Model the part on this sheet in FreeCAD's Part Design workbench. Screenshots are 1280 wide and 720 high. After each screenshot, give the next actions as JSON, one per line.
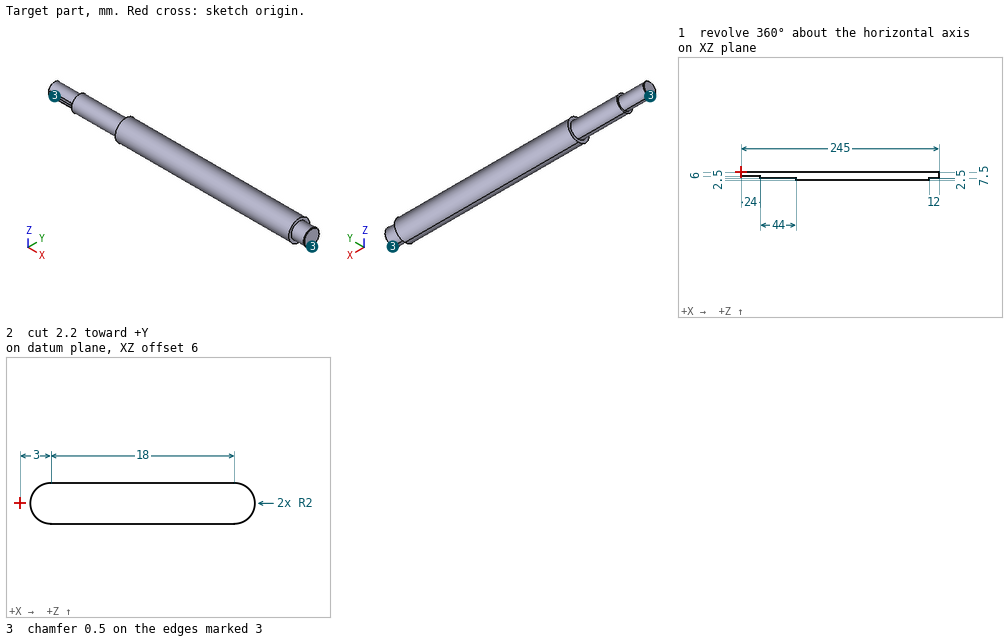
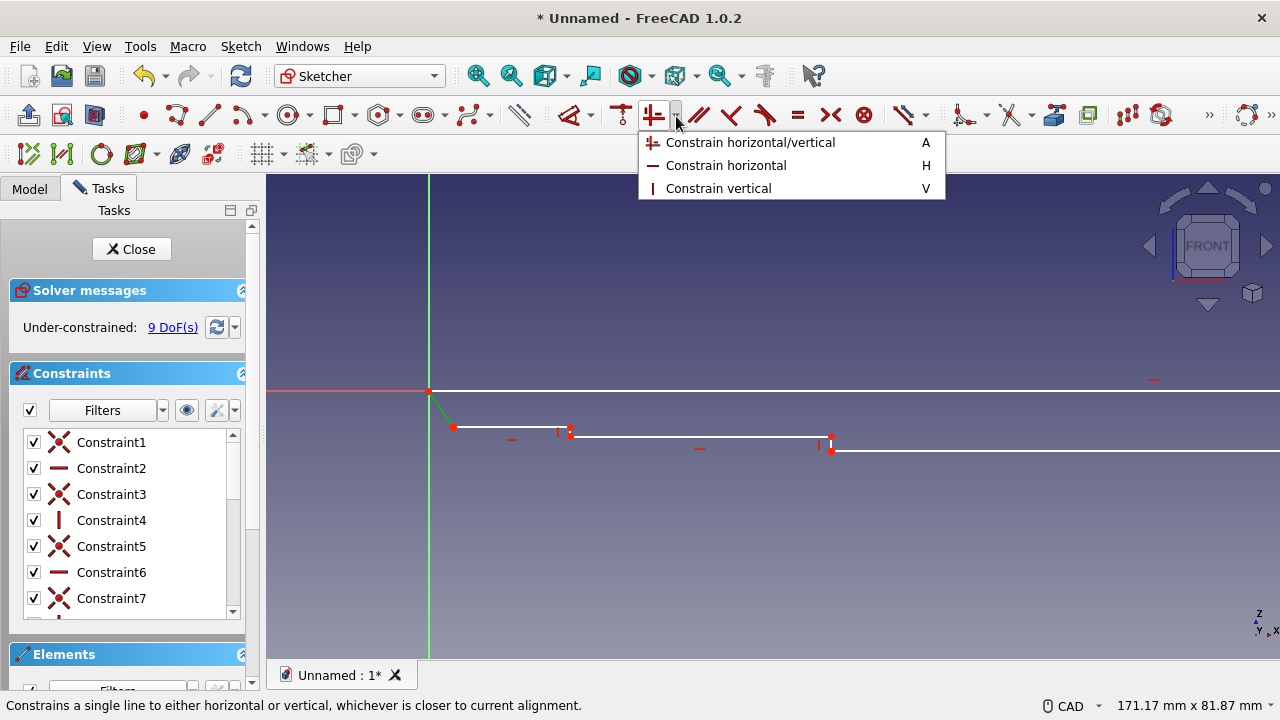
{"action": "left_click", "coordinate": [792, 188]}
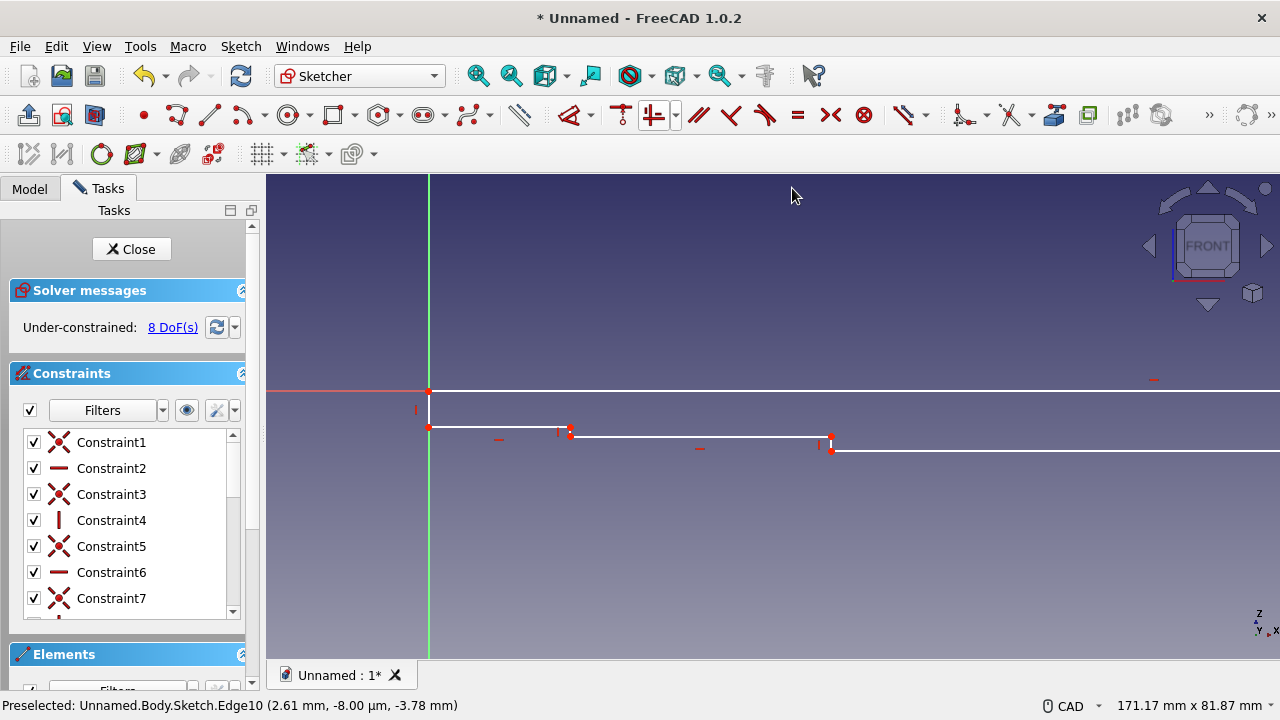
{"action": "scroll", "coordinate": [429, 417], "scroll_direction": "up", "scroll_amount": 2}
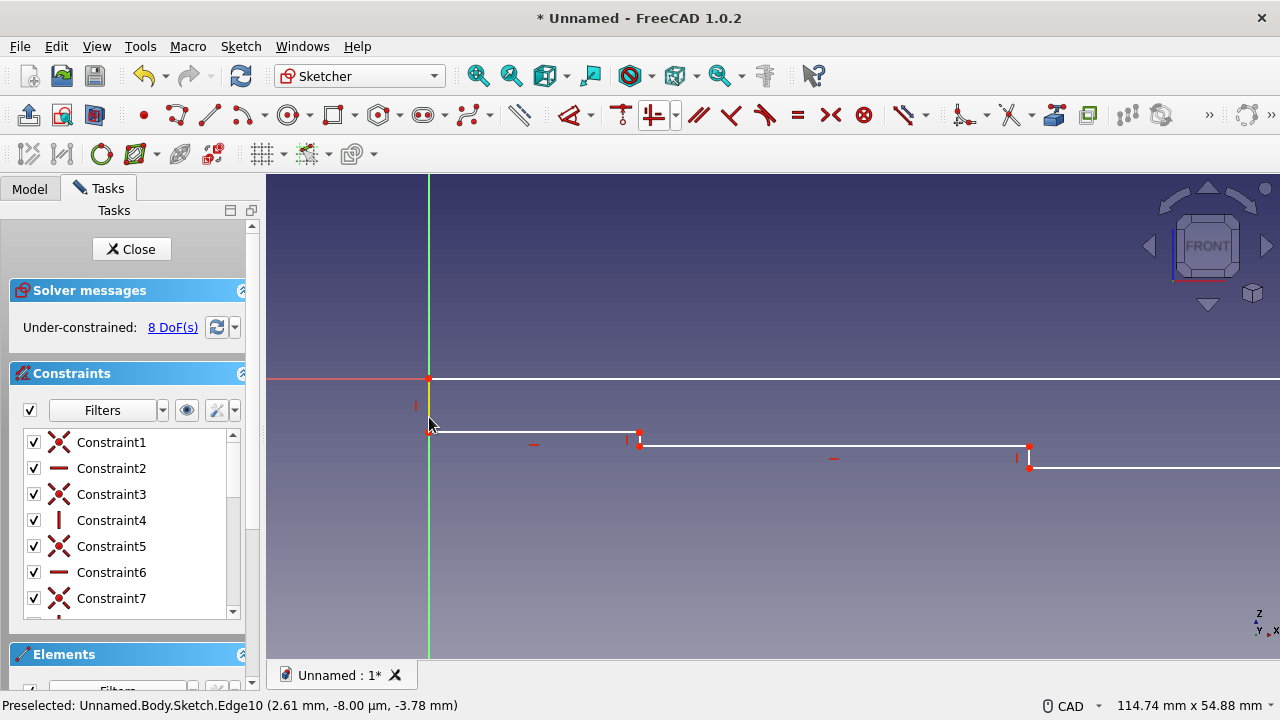
{"action": "left_click", "coordinate": [429, 416]}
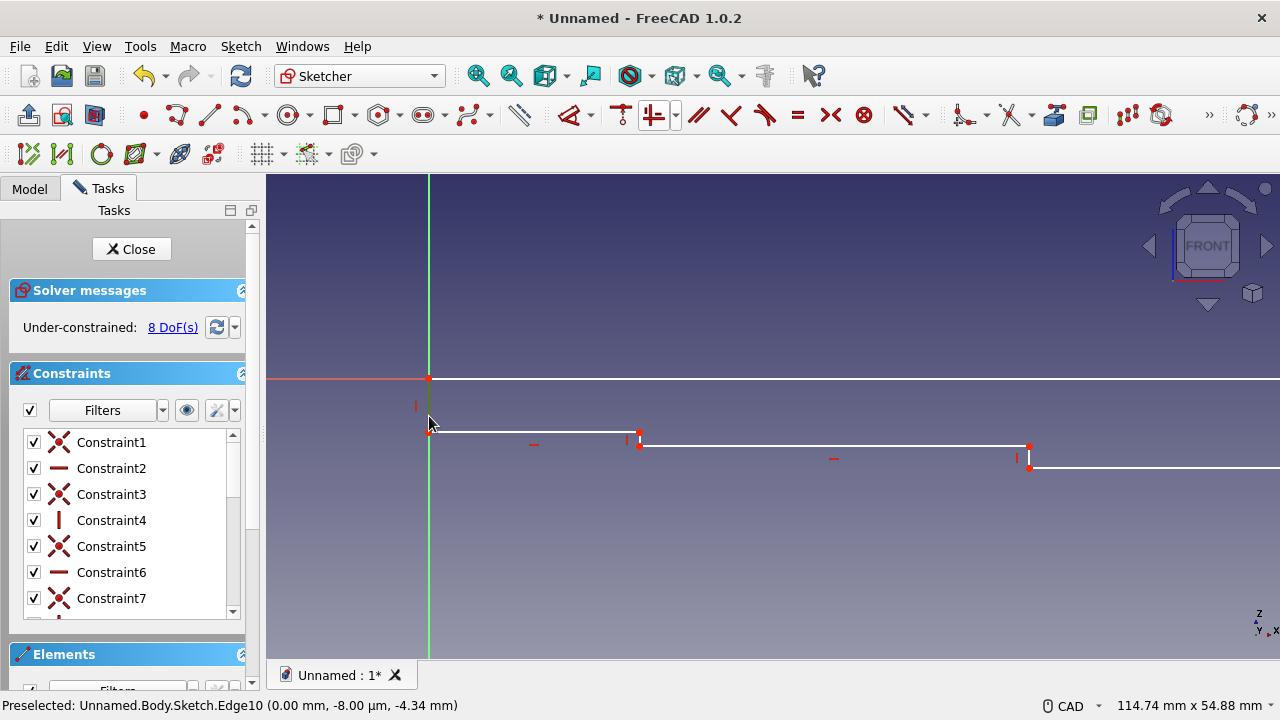
{"action": "key", "text": "i"}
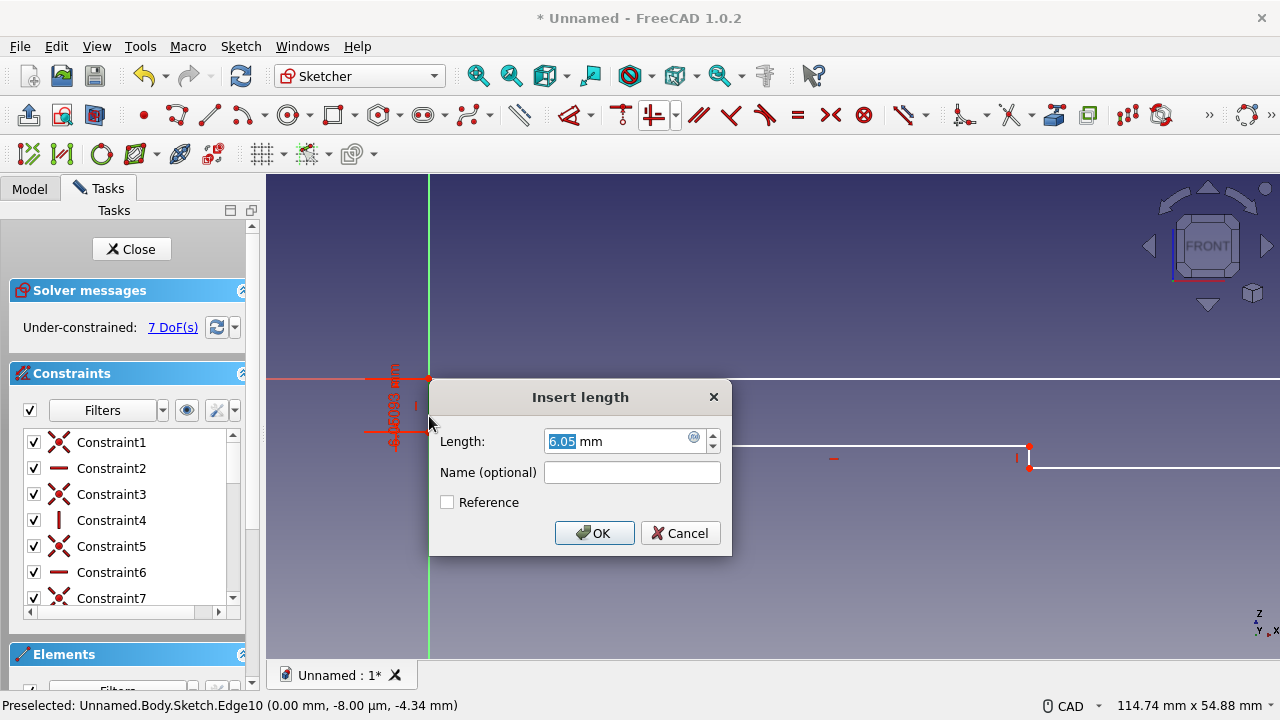
{"action": "type", "text": "6"}
{"action": "key", "text": "Return"}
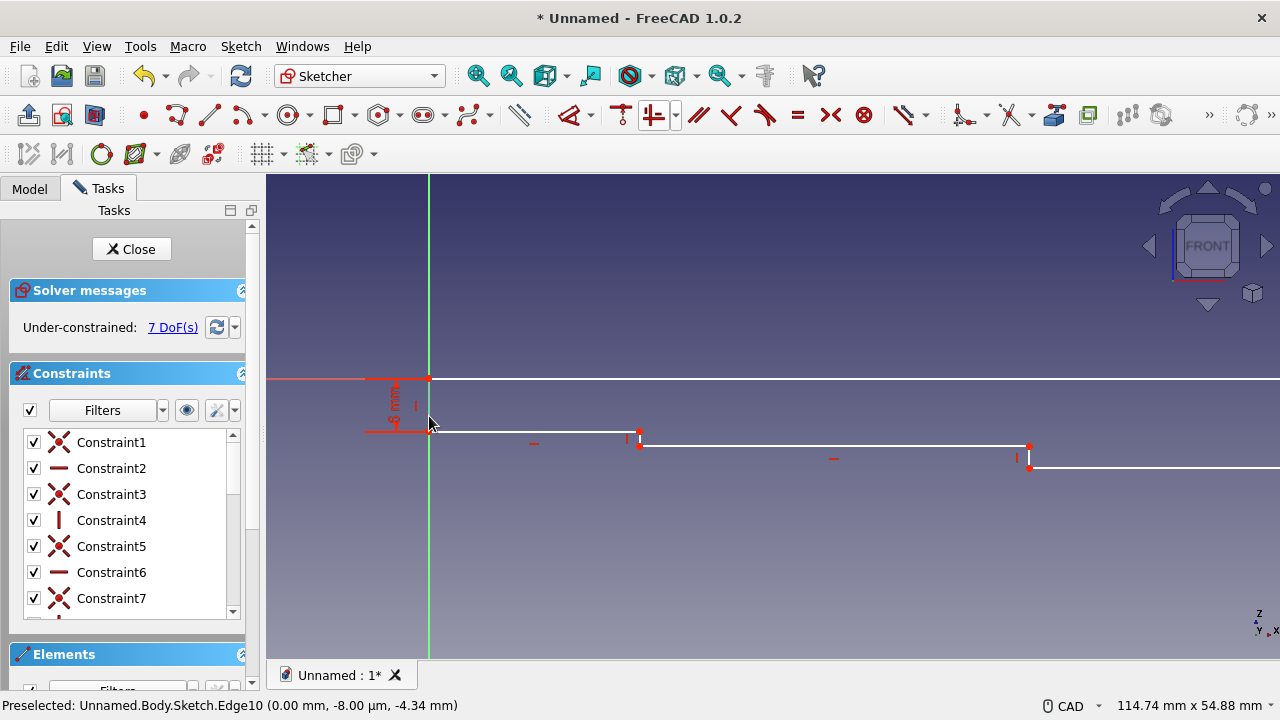
{"action": "scroll", "coordinate": [440, 414], "scroll_direction": "down", "scroll_amount": 7}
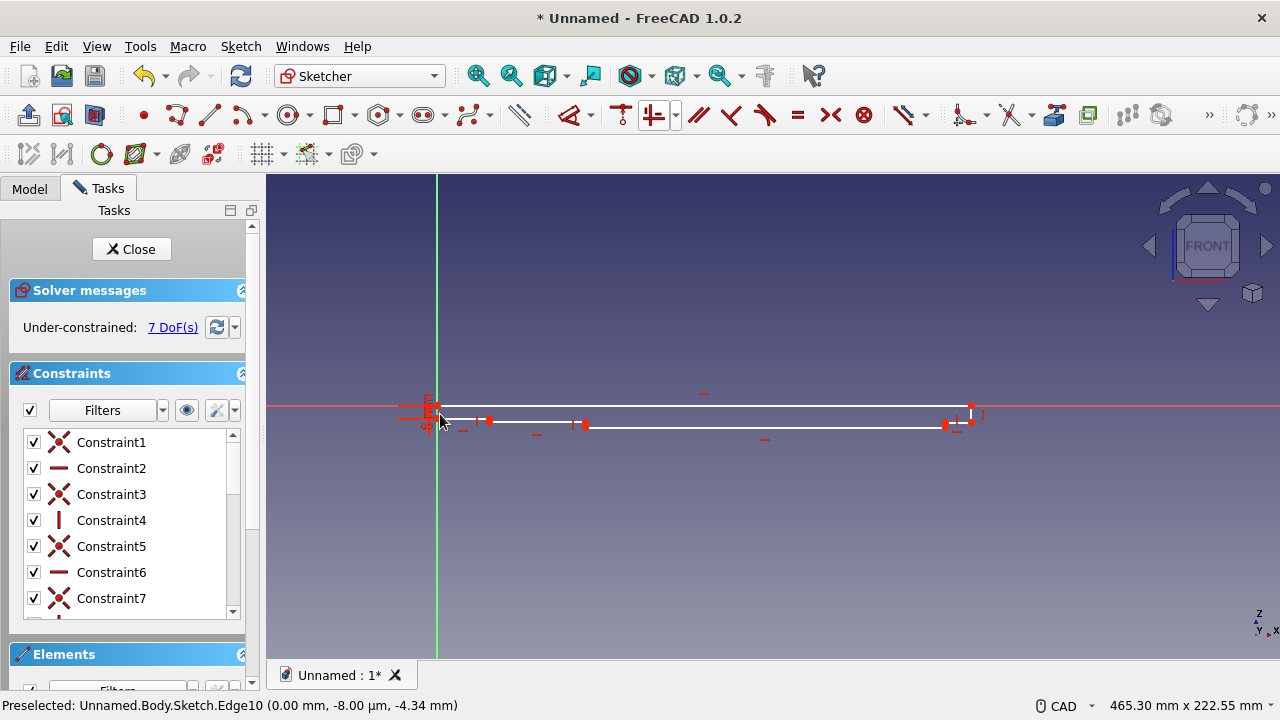
{"action": "scroll", "coordinate": [963, 423], "scroll_direction": "up", "scroll_amount": 3}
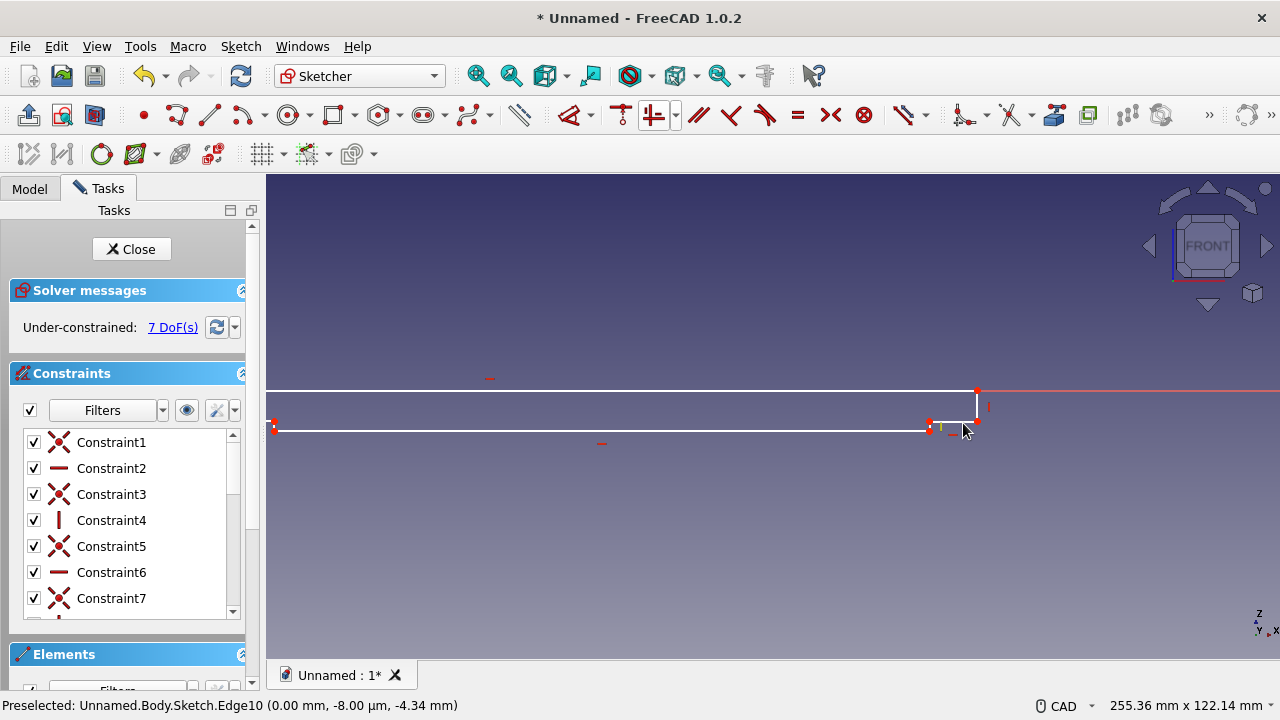
{"action": "left_click", "coordinate": [963, 422]}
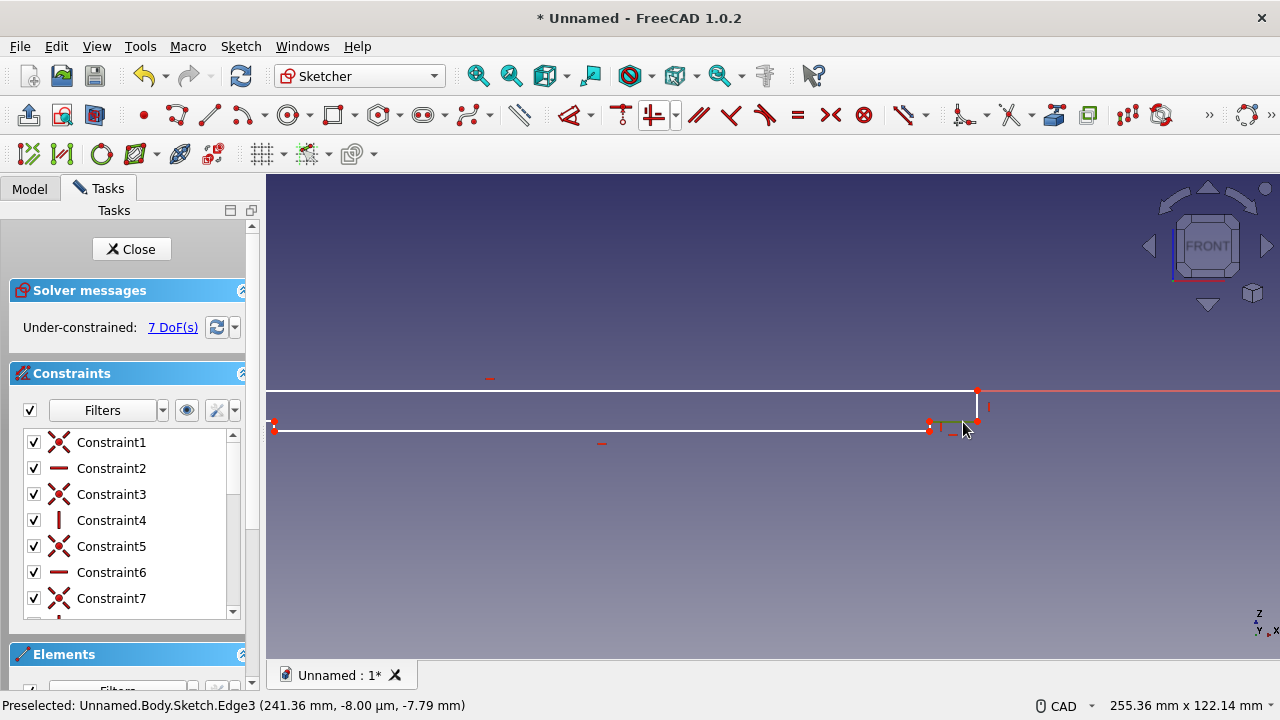
{"action": "key", "text": "l"}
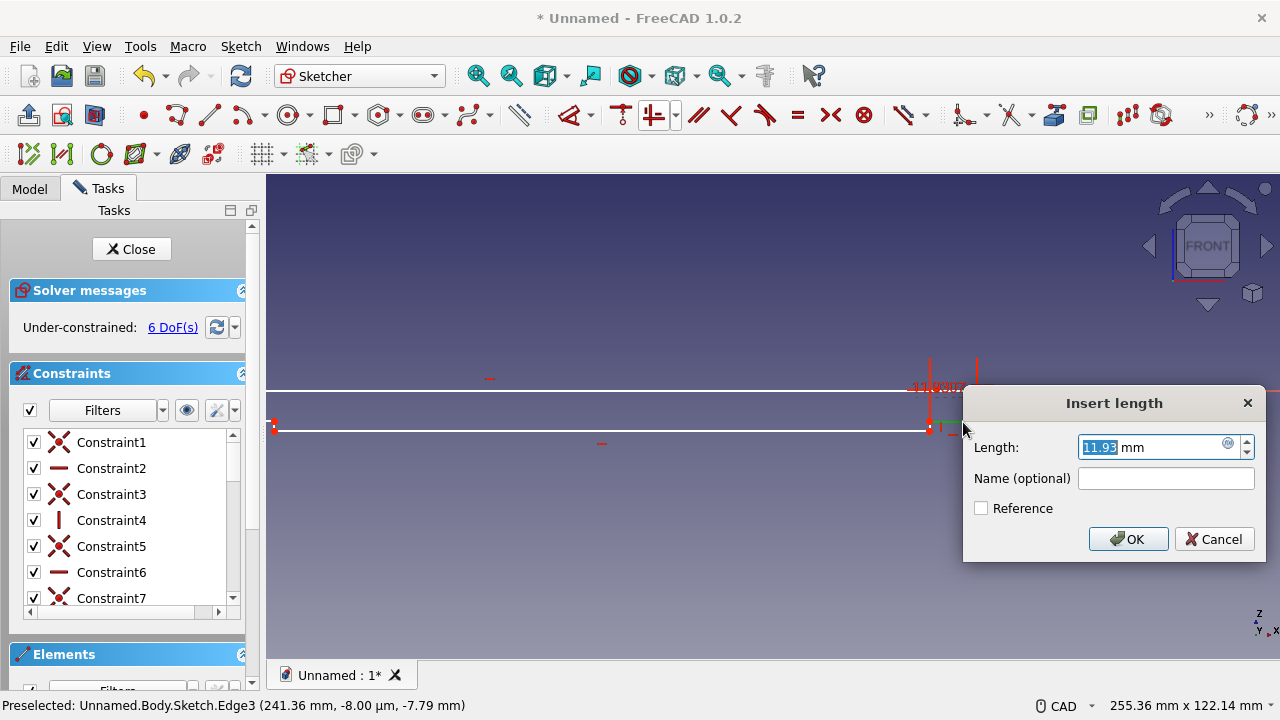
{"action": "type", "text": "12"}
{"action": "key", "text": "Return"}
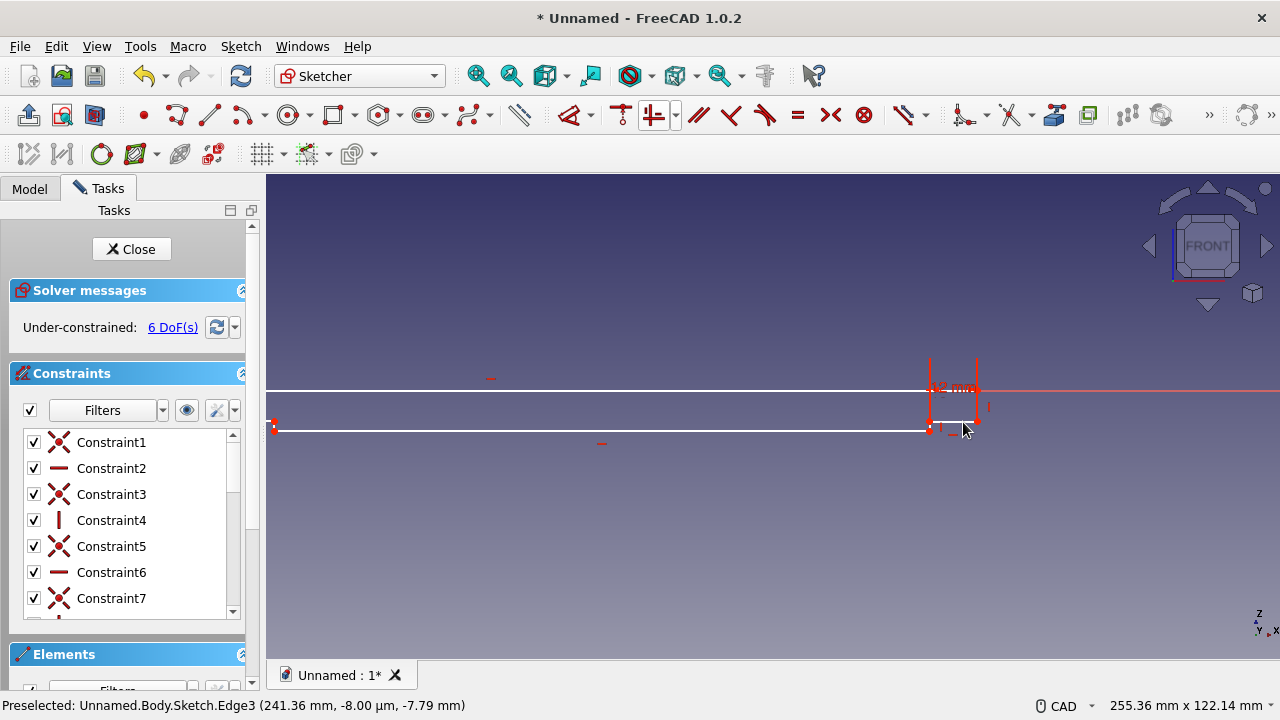
{"action": "scroll", "coordinate": [964, 423], "scroll_direction": "down", "scroll_amount": 3}